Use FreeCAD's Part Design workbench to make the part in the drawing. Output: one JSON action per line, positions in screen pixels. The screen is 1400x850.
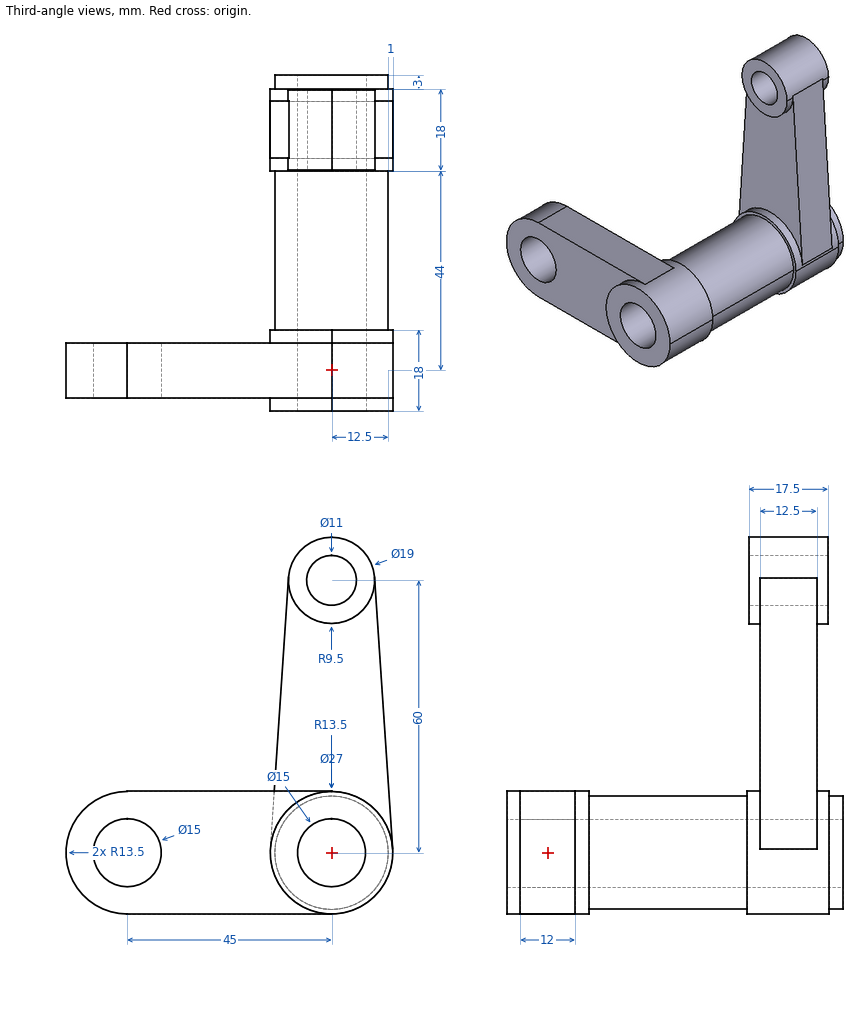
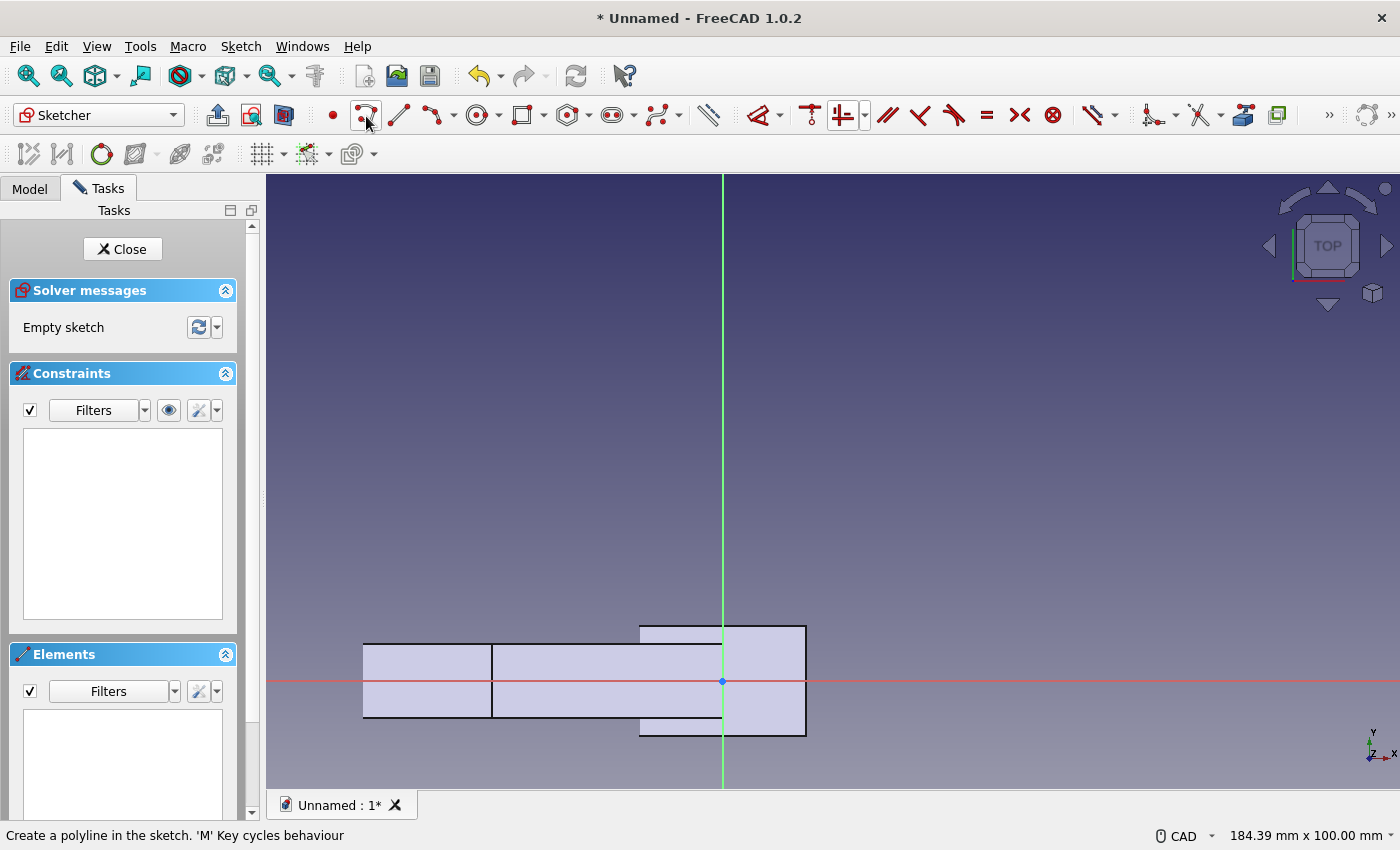
{"action": "left_click", "coordinate": [723, 681]}
{"action": "left_click", "coordinate": [800, 672]}
{"action": "left_click", "coordinate": [800, 410]}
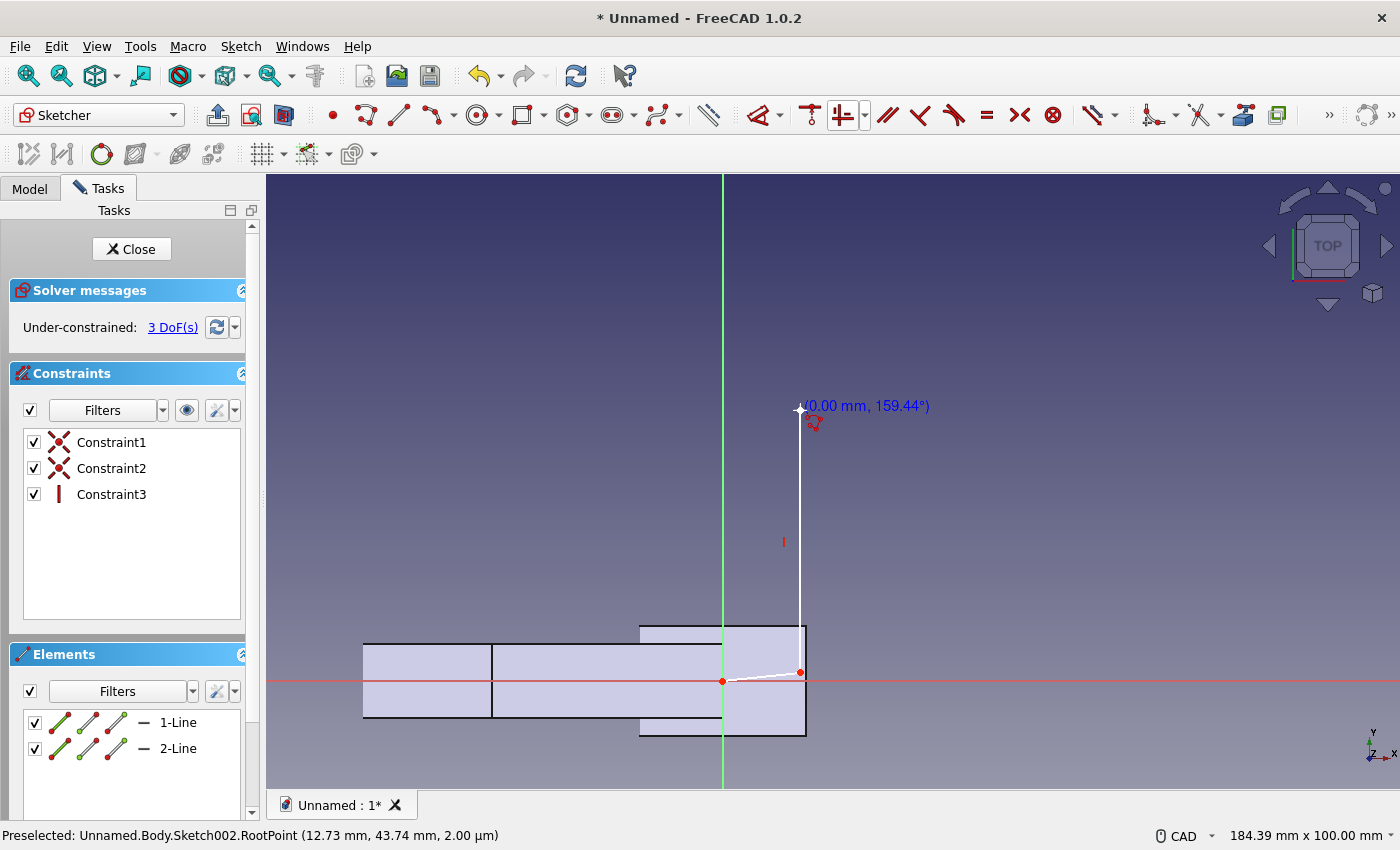
{"action": "scroll", "coordinate": [806, 410], "scroll_direction": "up", "scroll_amount": 5}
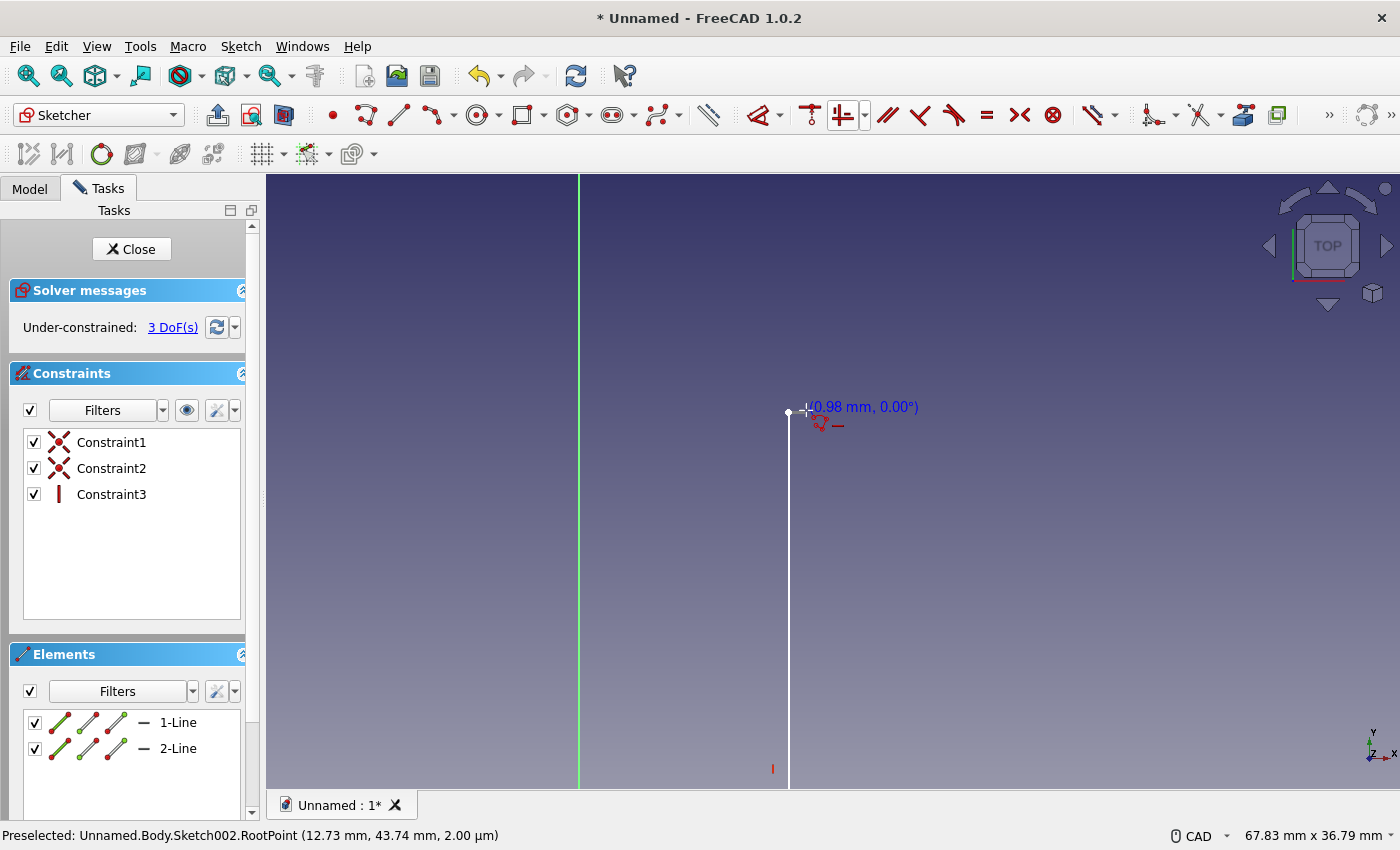
{"action": "left_click", "coordinate": [805, 409]}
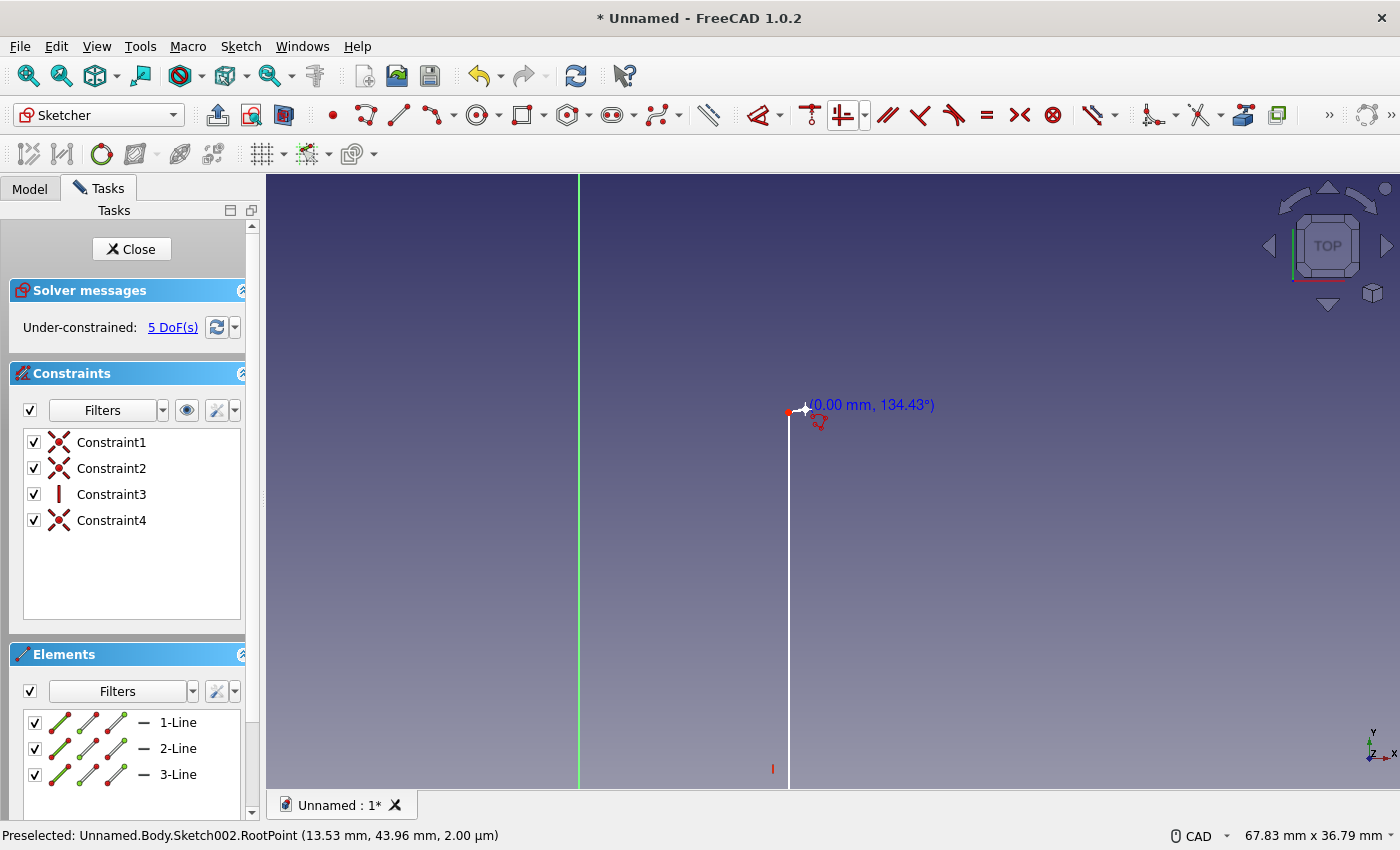
{"action": "scroll", "coordinate": [807, 411], "scroll_direction": "down", "scroll_amount": 5}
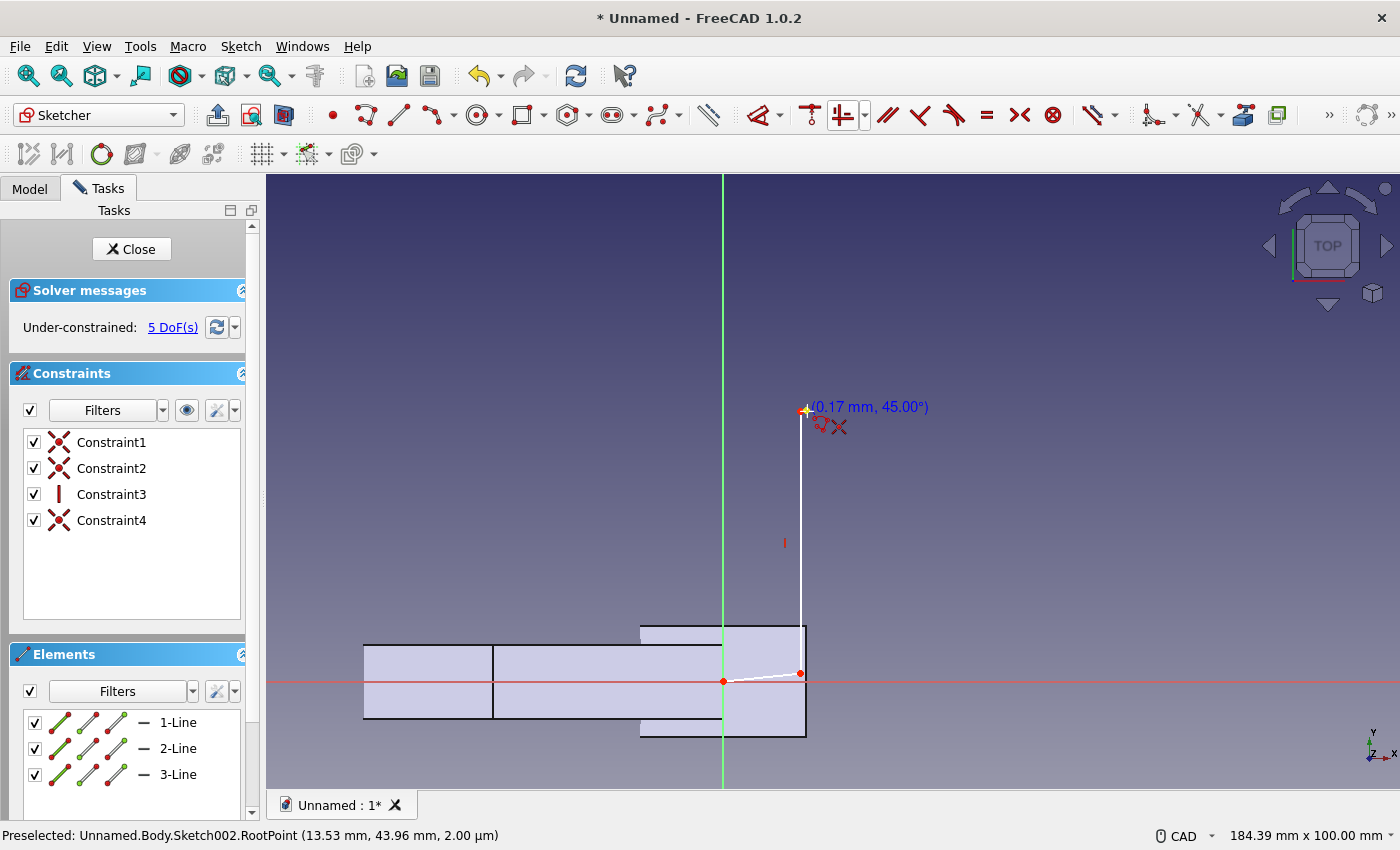
{"action": "left_click", "coordinate": [807, 300]}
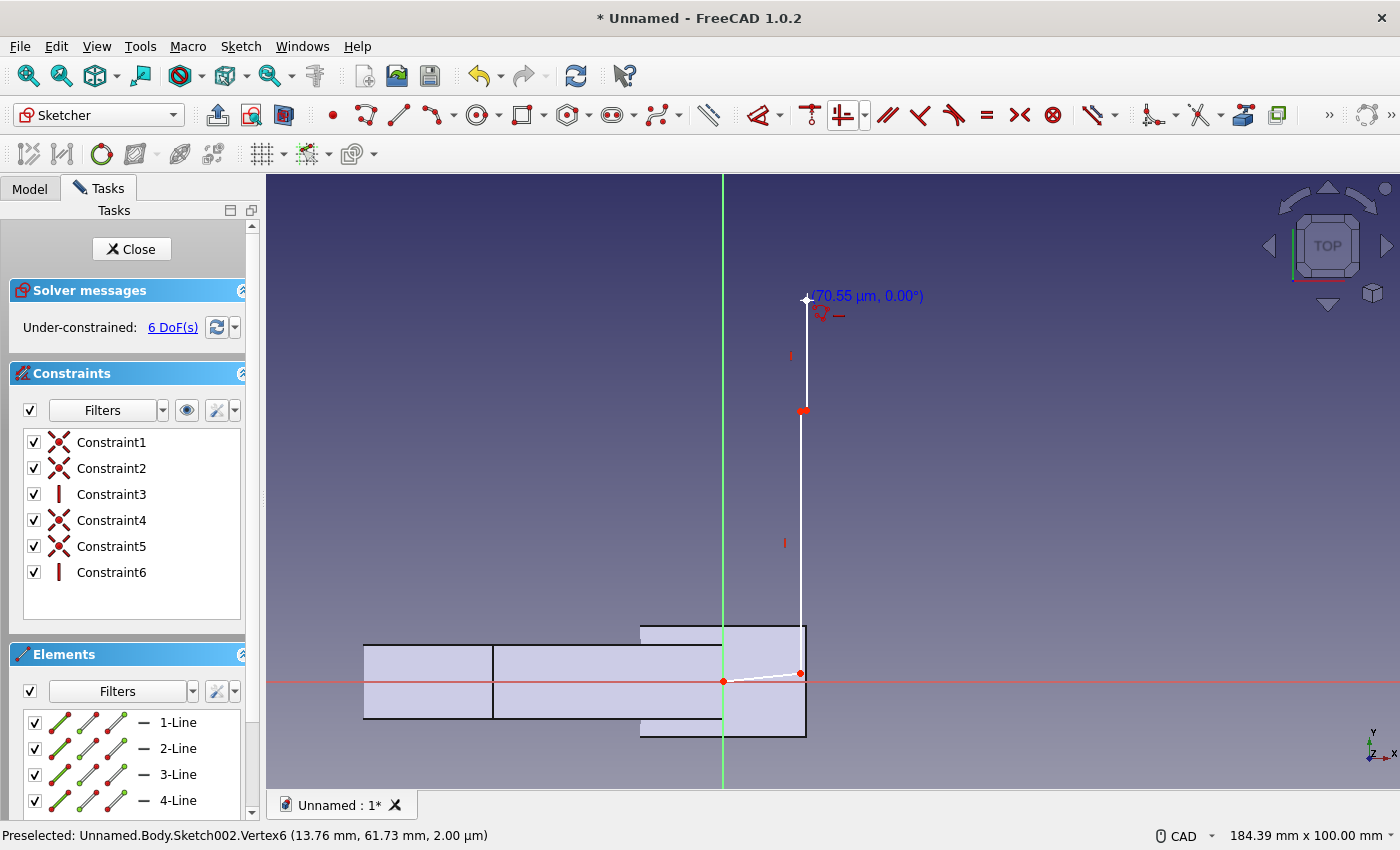
{"action": "scroll", "coordinate": [800, 300], "scroll_direction": "up", "scroll_amount": 5}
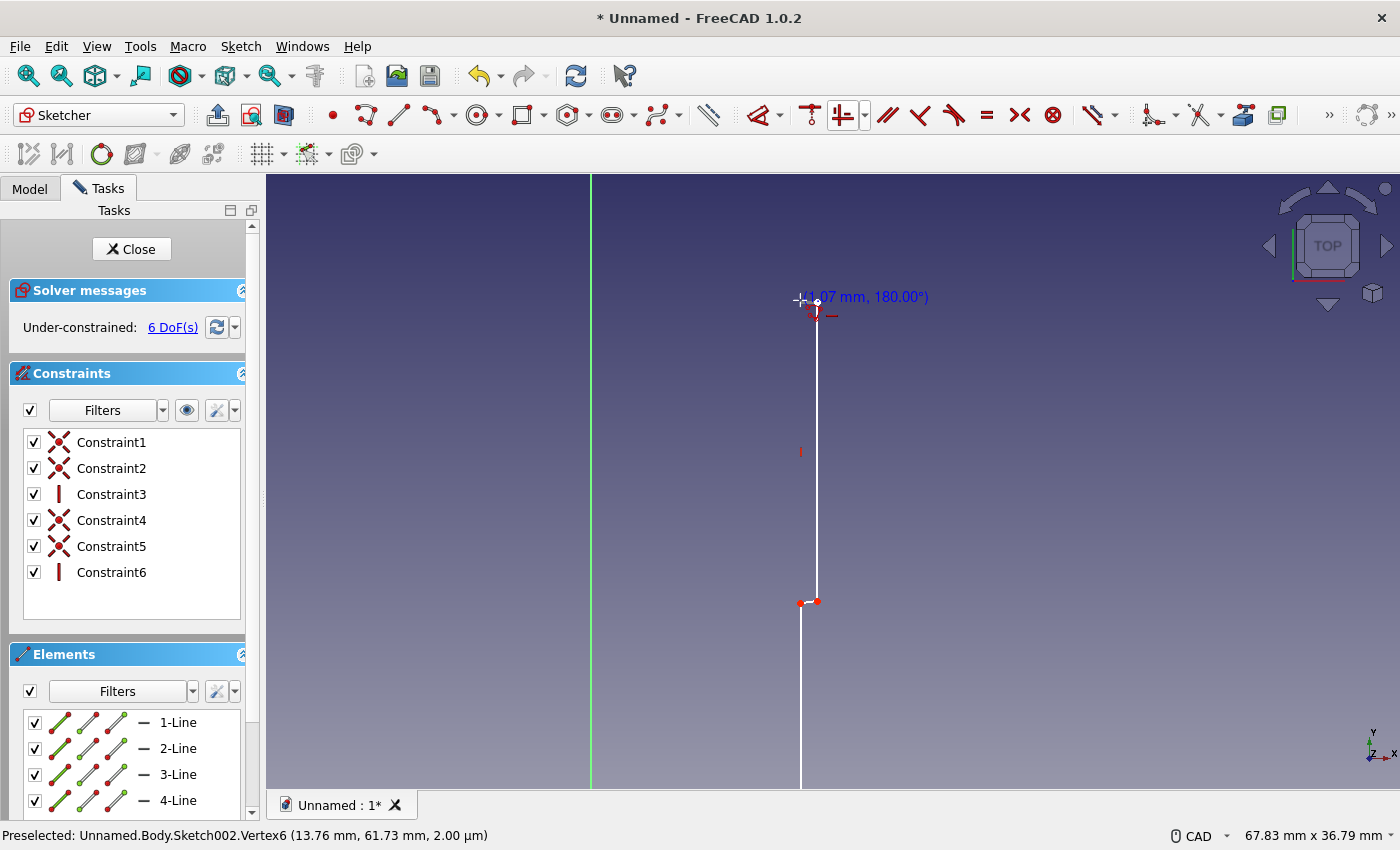
{"action": "left_click", "coordinate": [800, 300]}
{"action": "left_click", "coordinate": [800, 250]}
{"action": "left_click", "coordinate": [600, 250]}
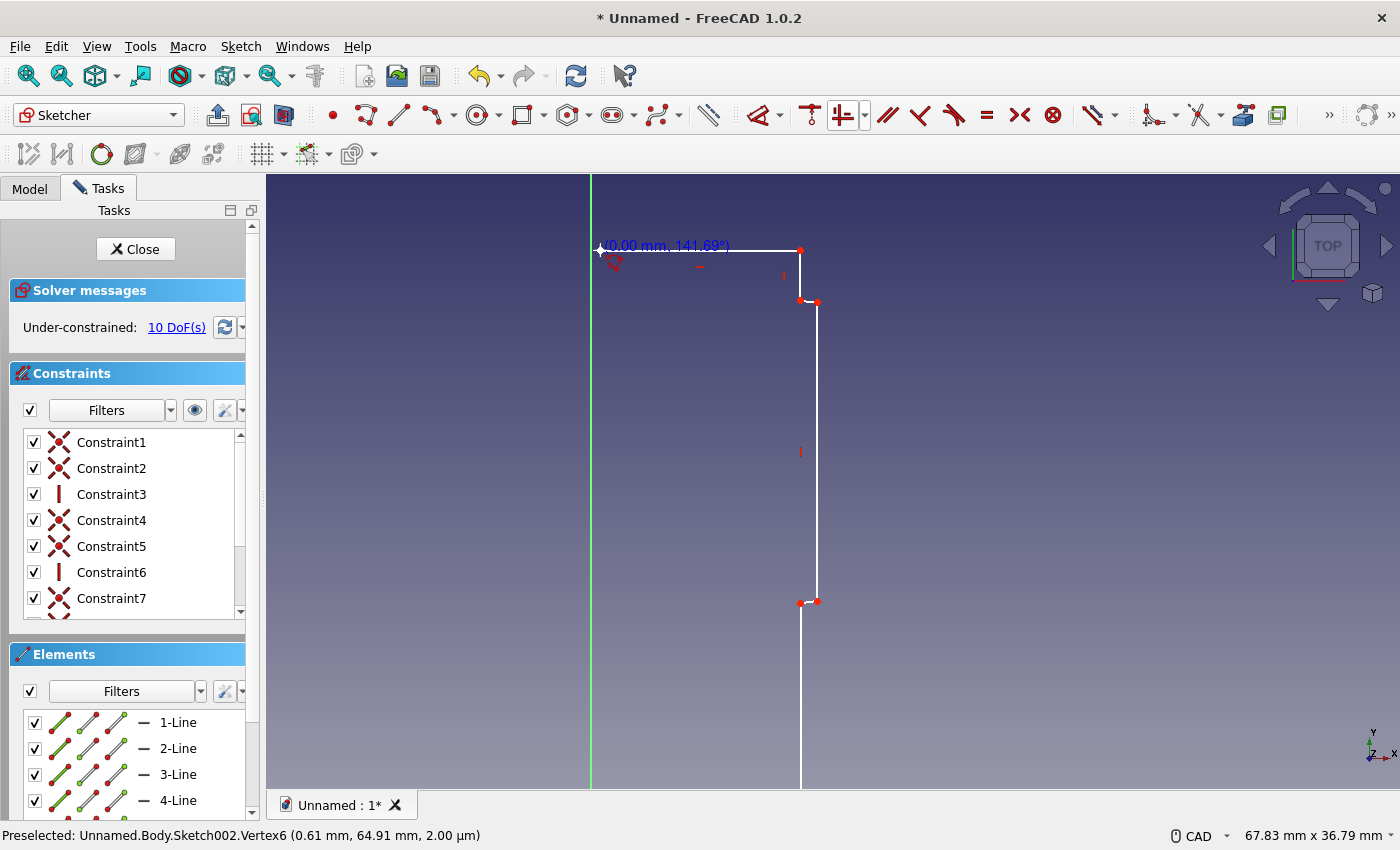
{"action": "scroll", "coordinate": [800, 300], "scroll_direction": "down", "scroll_amount": 5}